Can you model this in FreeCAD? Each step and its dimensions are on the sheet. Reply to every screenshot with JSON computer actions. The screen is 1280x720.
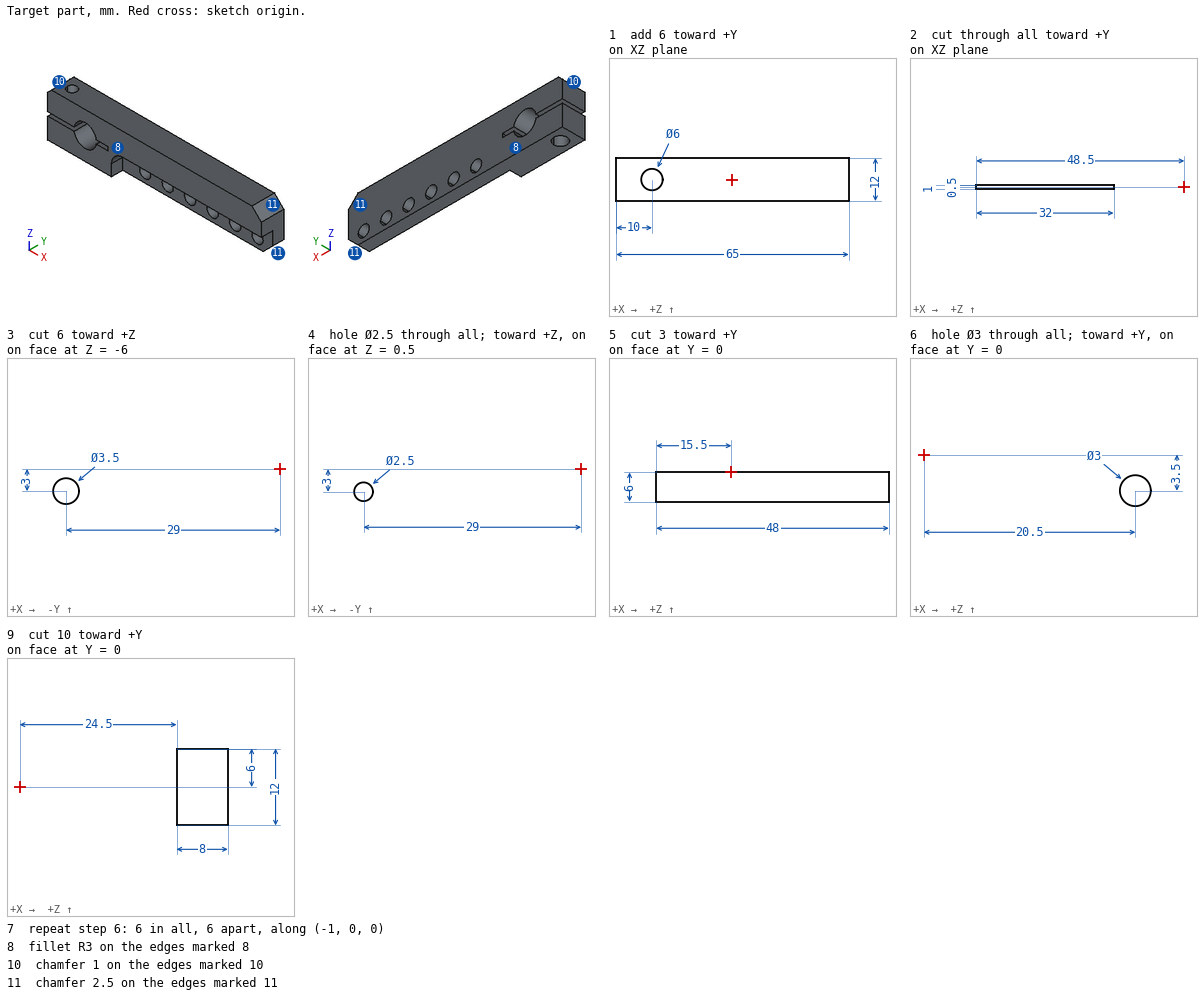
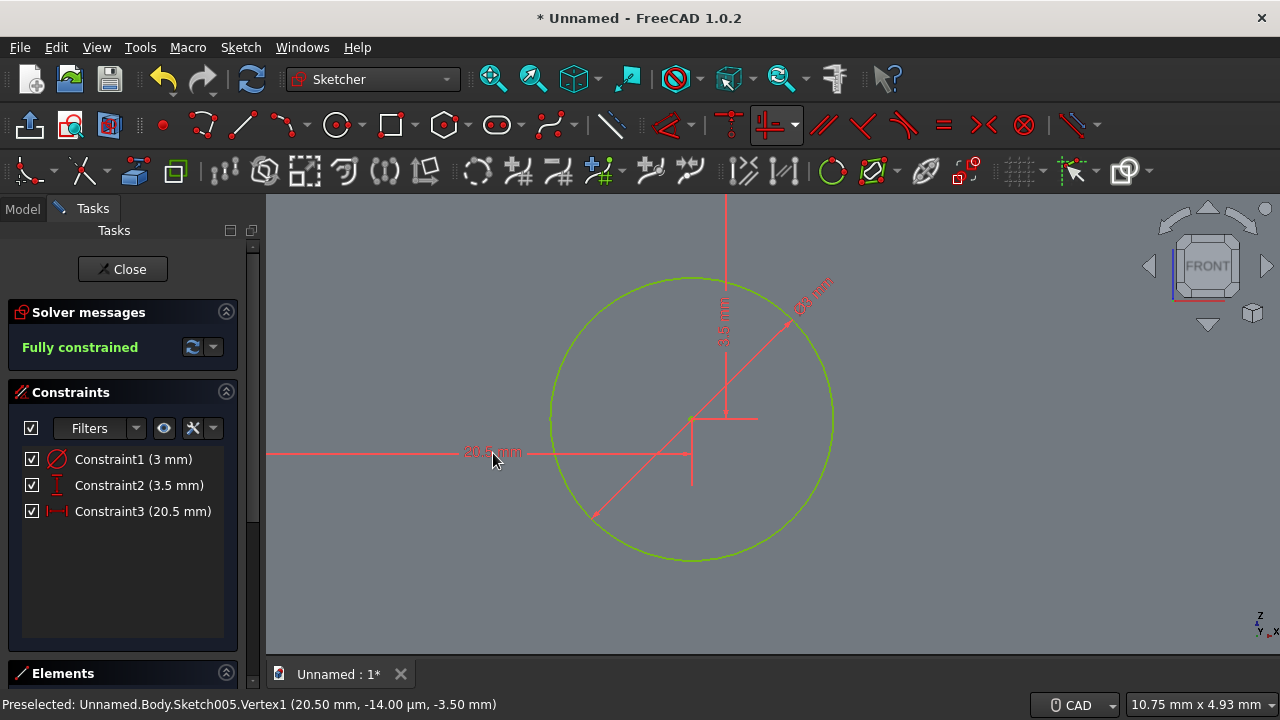
{"action": "left_click", "coordinate": [123, 269]}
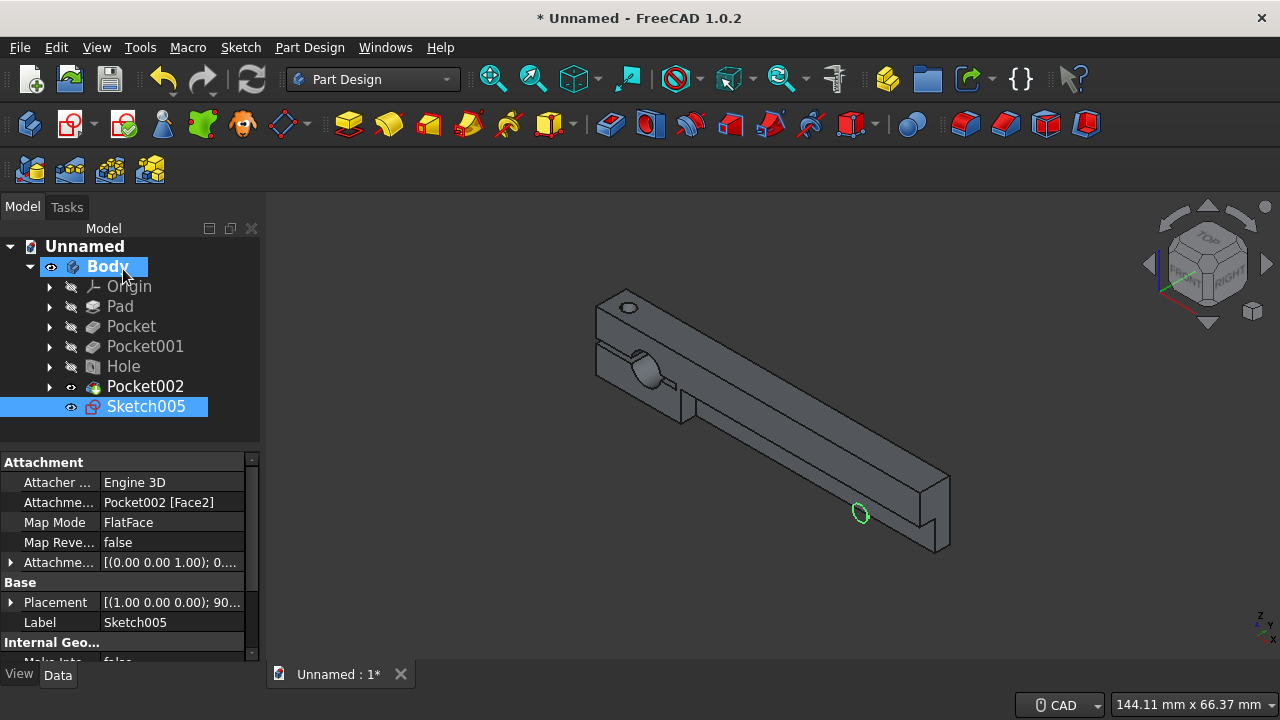
{"action": "left_click", "coordinate": [652, 124]}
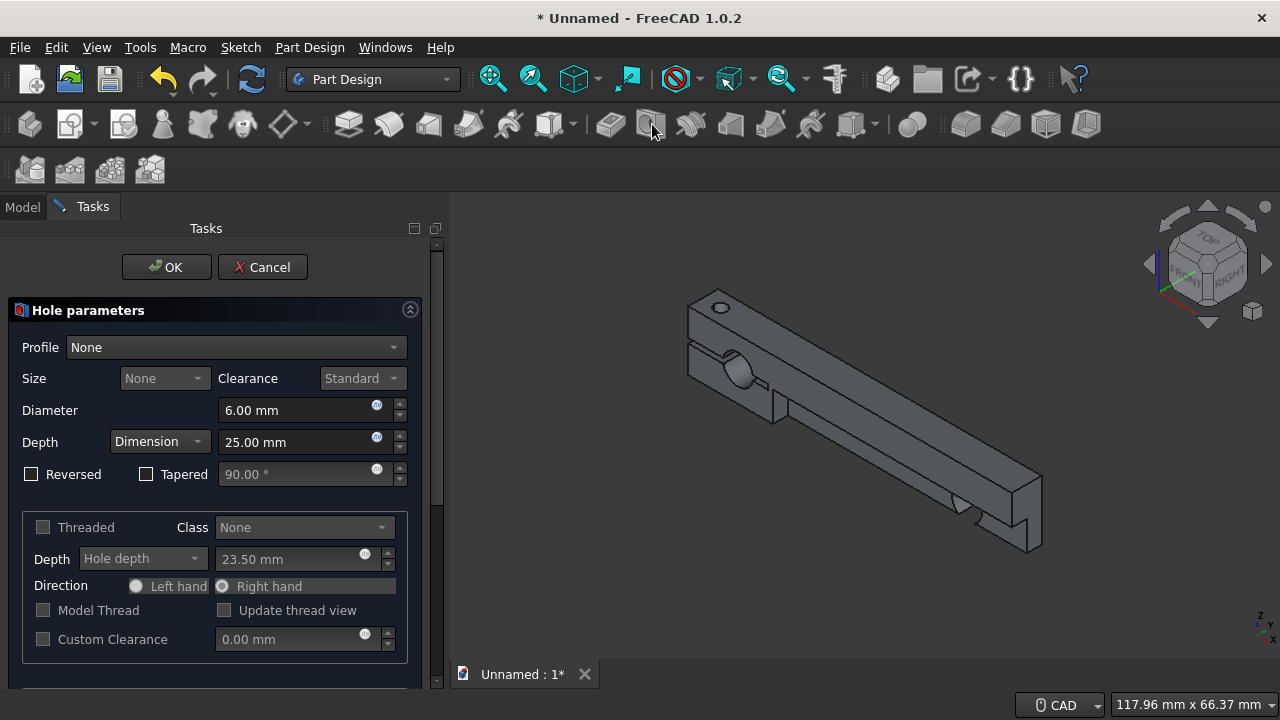
{"action": "triple_click", "coordinate": [305, 410]}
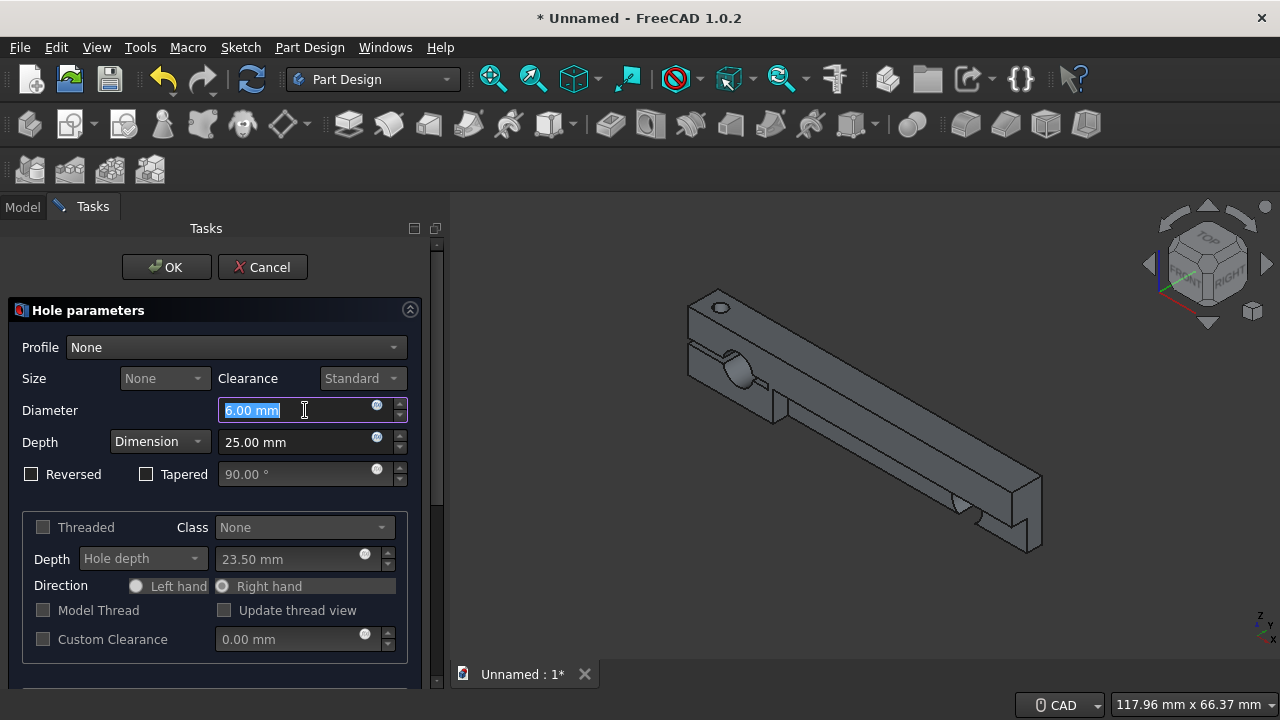
{"action": "type", "text": "3"}
{"action": "key", "text": "Tab"}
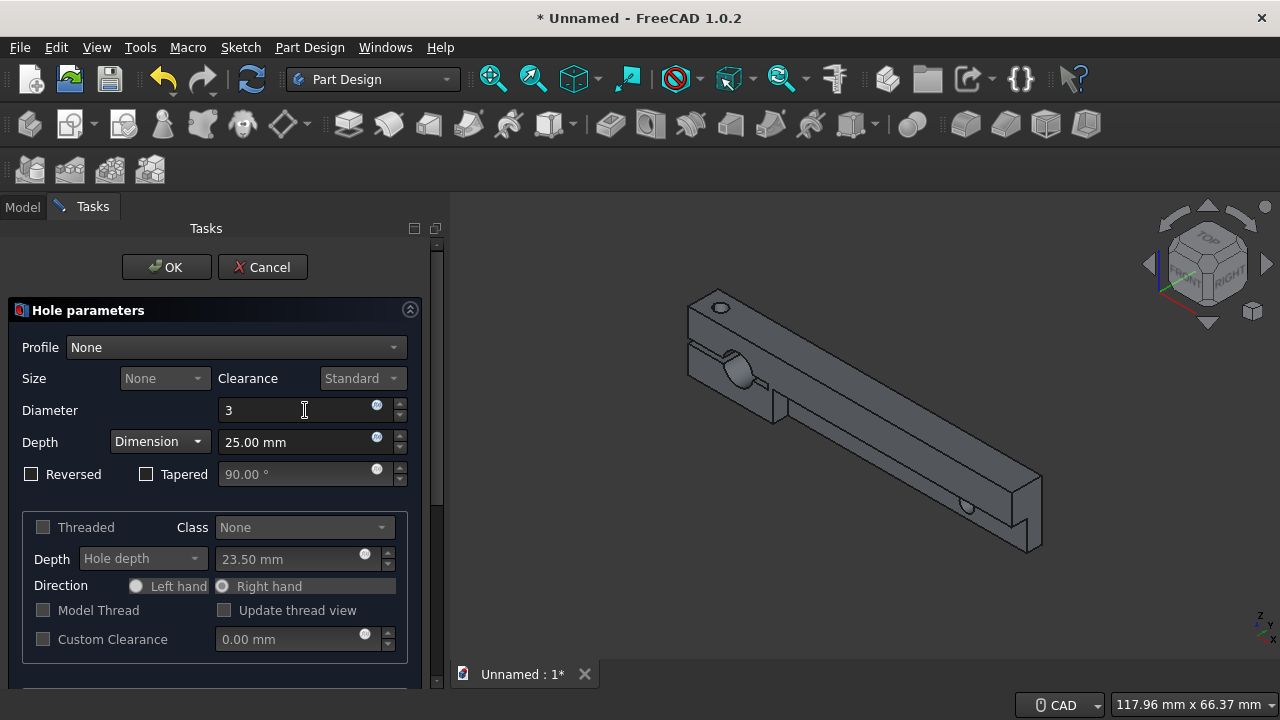
{"action": "left_click", "coordinate": [161, 442]}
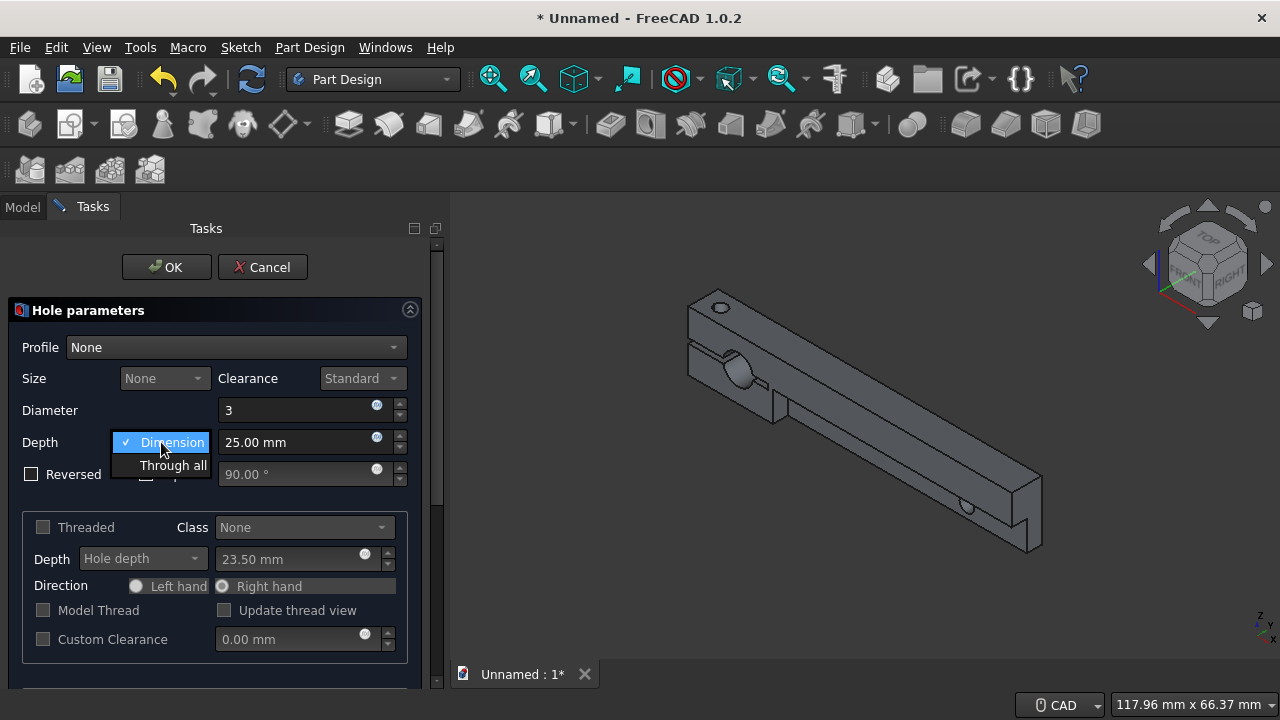
{"action": "left_click", "coordinate": [160, 466]}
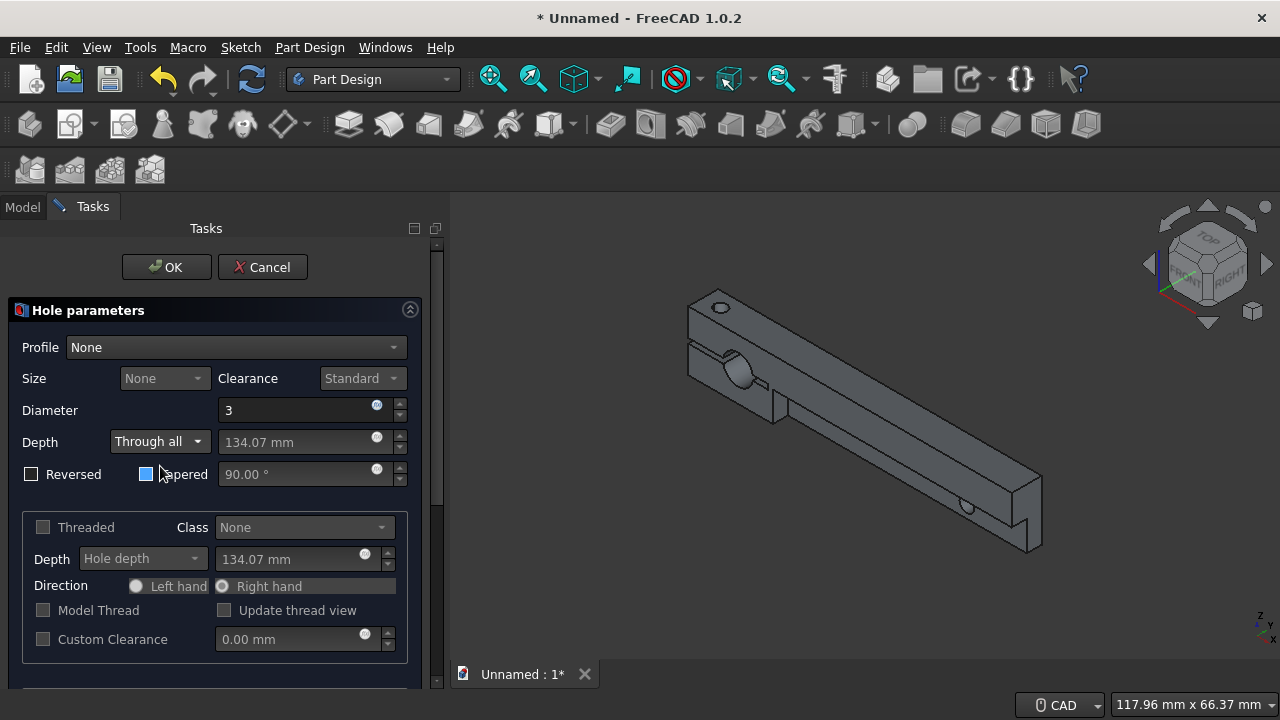
{"action": "left_click", "coordinate": [167, 267]}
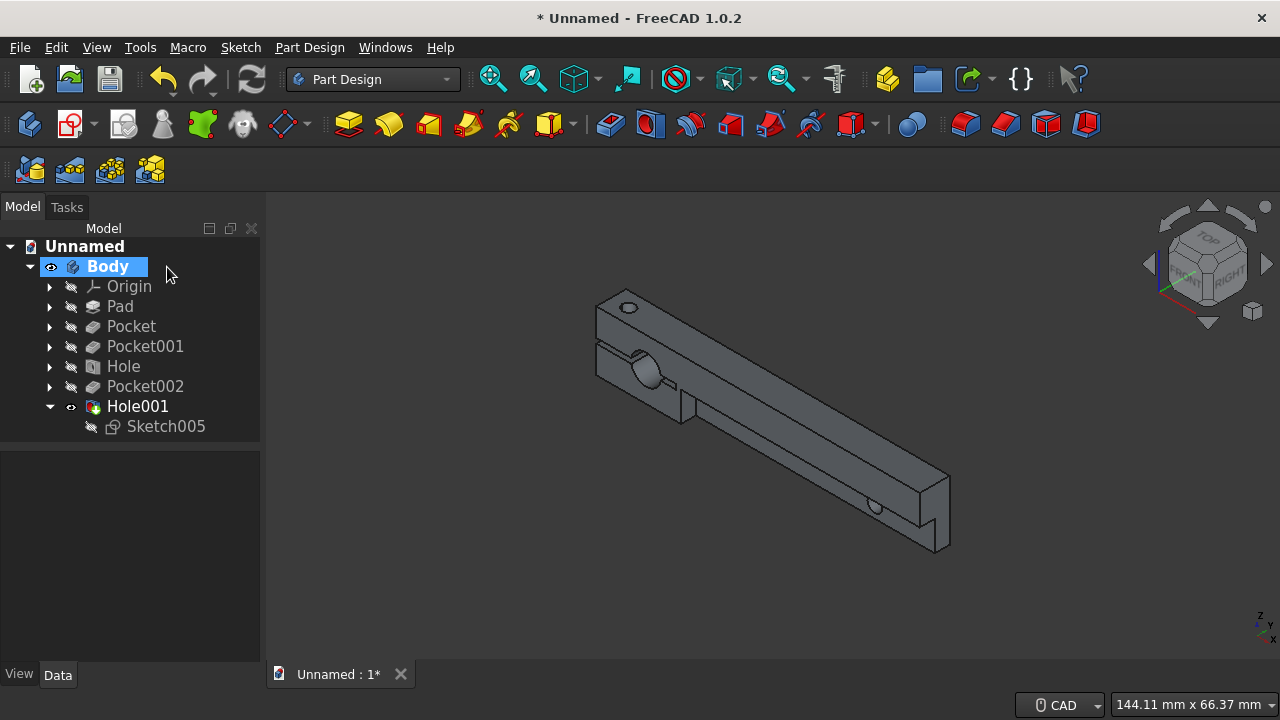
{"action": "left_click", "coordinate": [116, 407]}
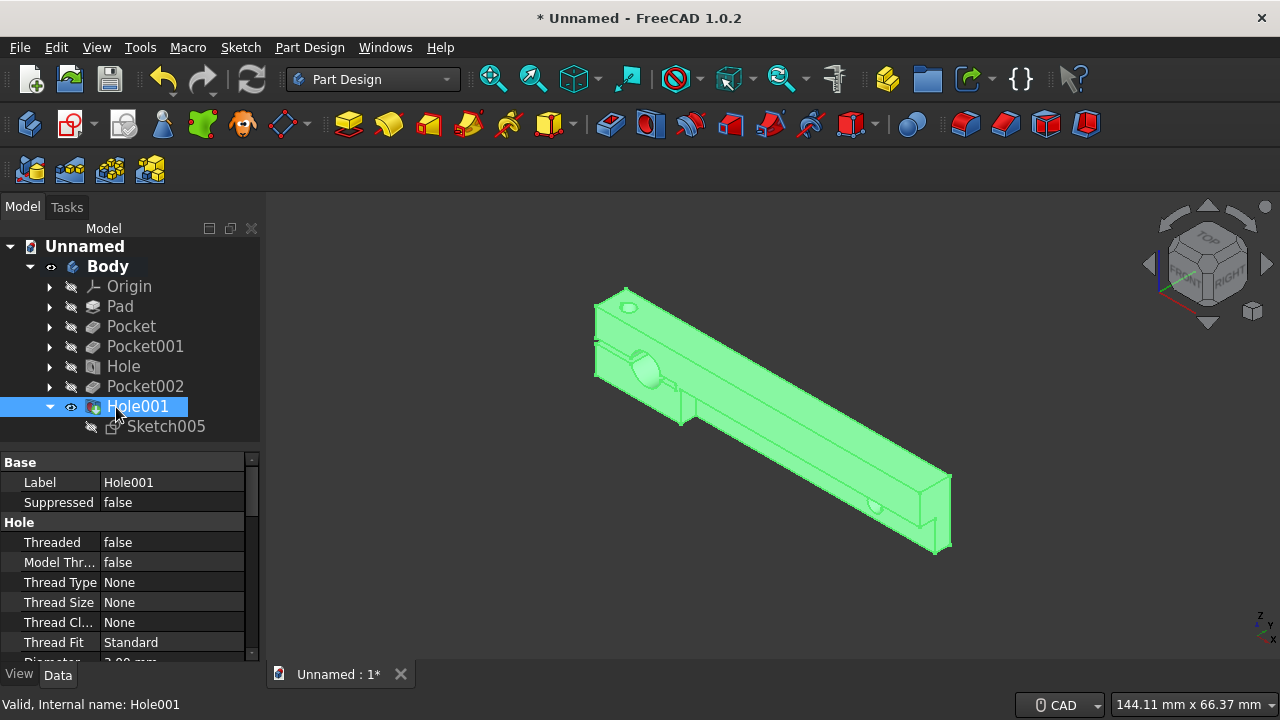
{"action": "left_click", "coordinate": [70, 170]}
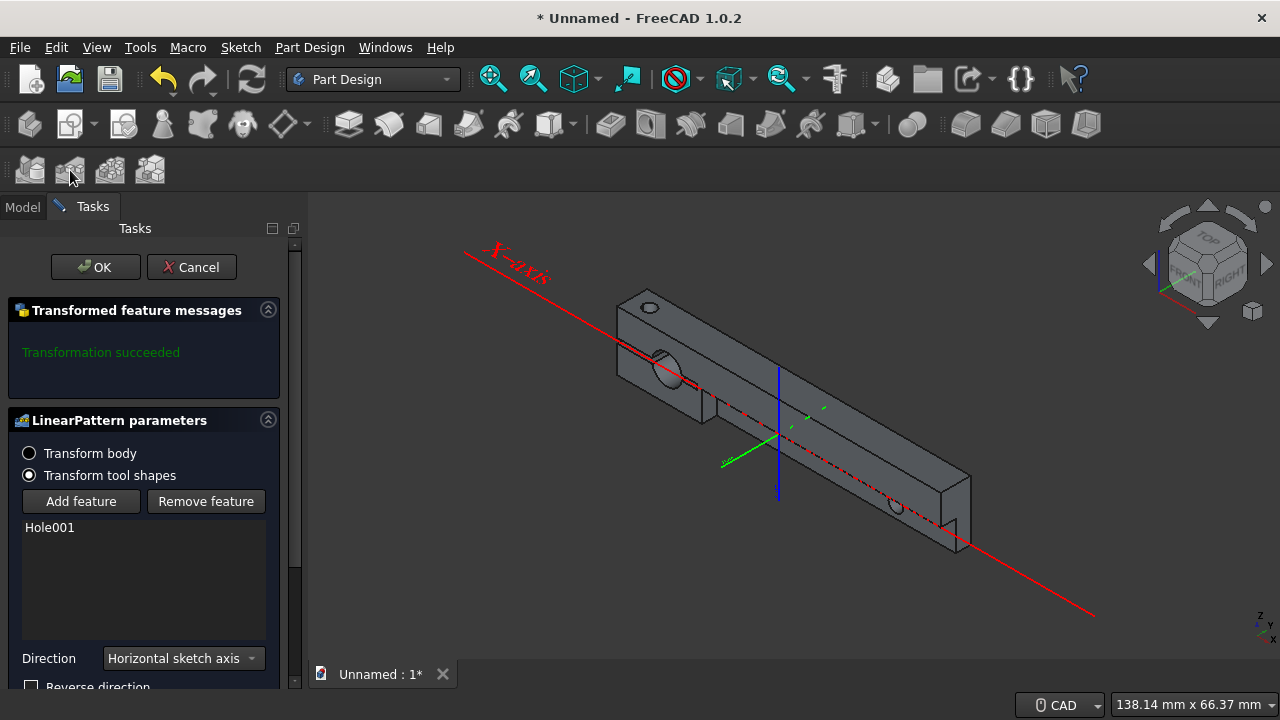
{"action": "left_click", "coordinate": [184, 658]}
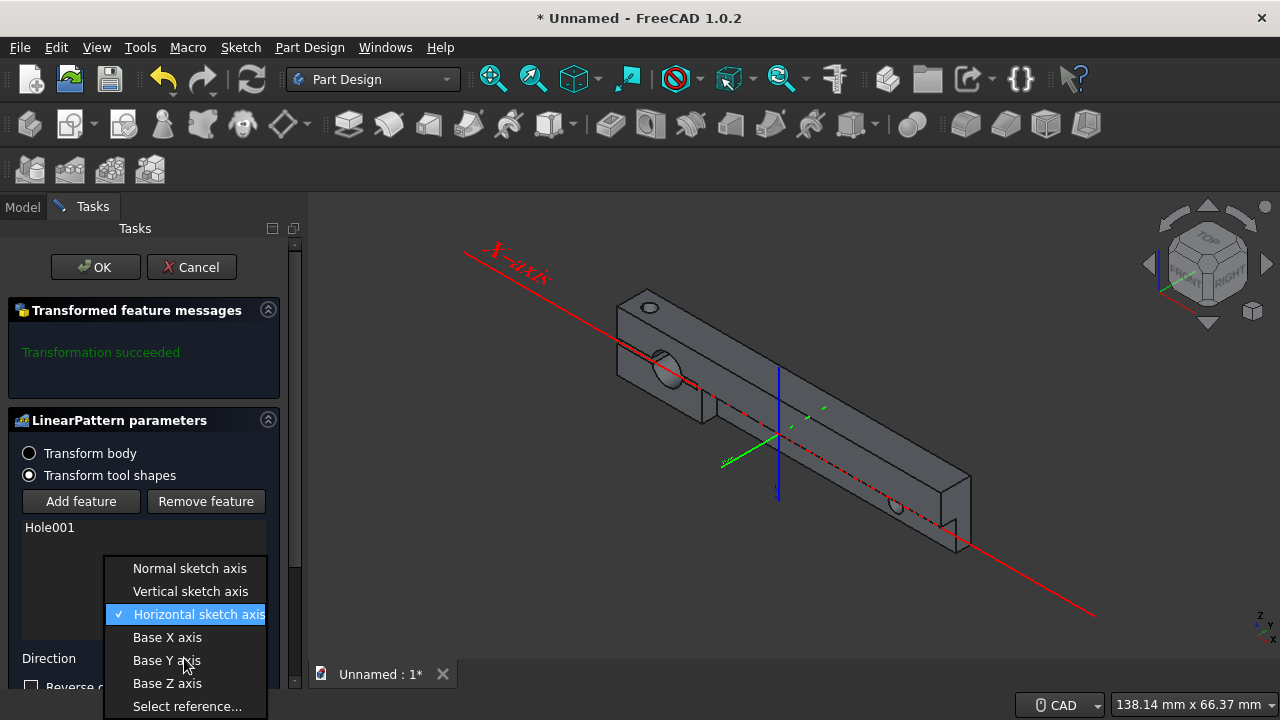
{"action": "left_click", "coordinate": [184, 638]}